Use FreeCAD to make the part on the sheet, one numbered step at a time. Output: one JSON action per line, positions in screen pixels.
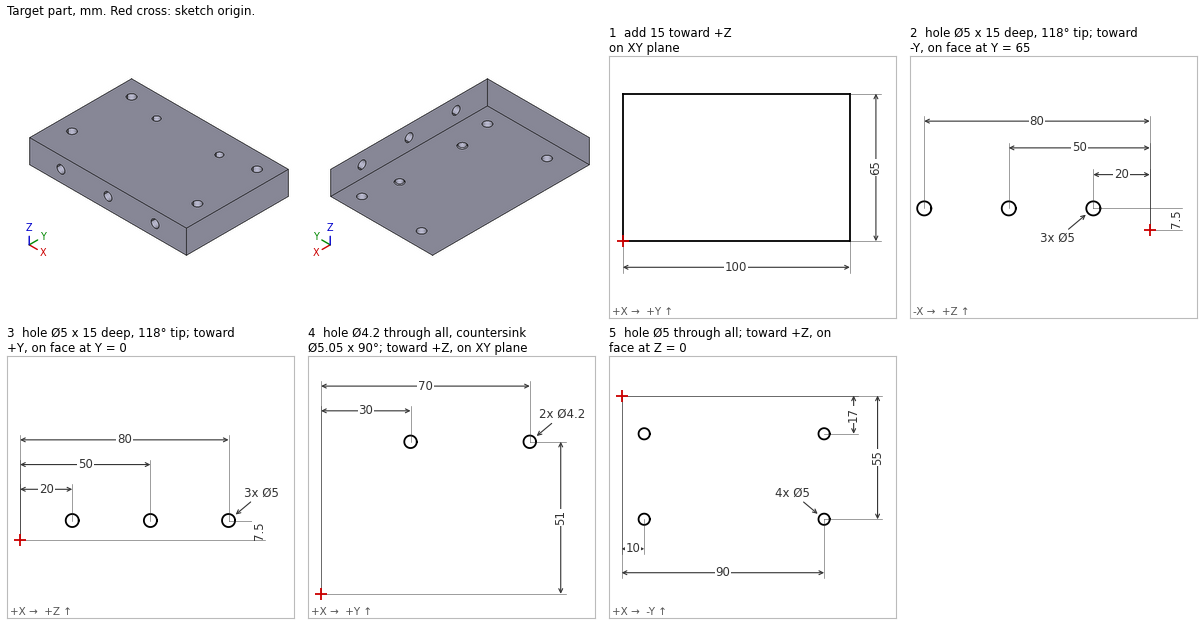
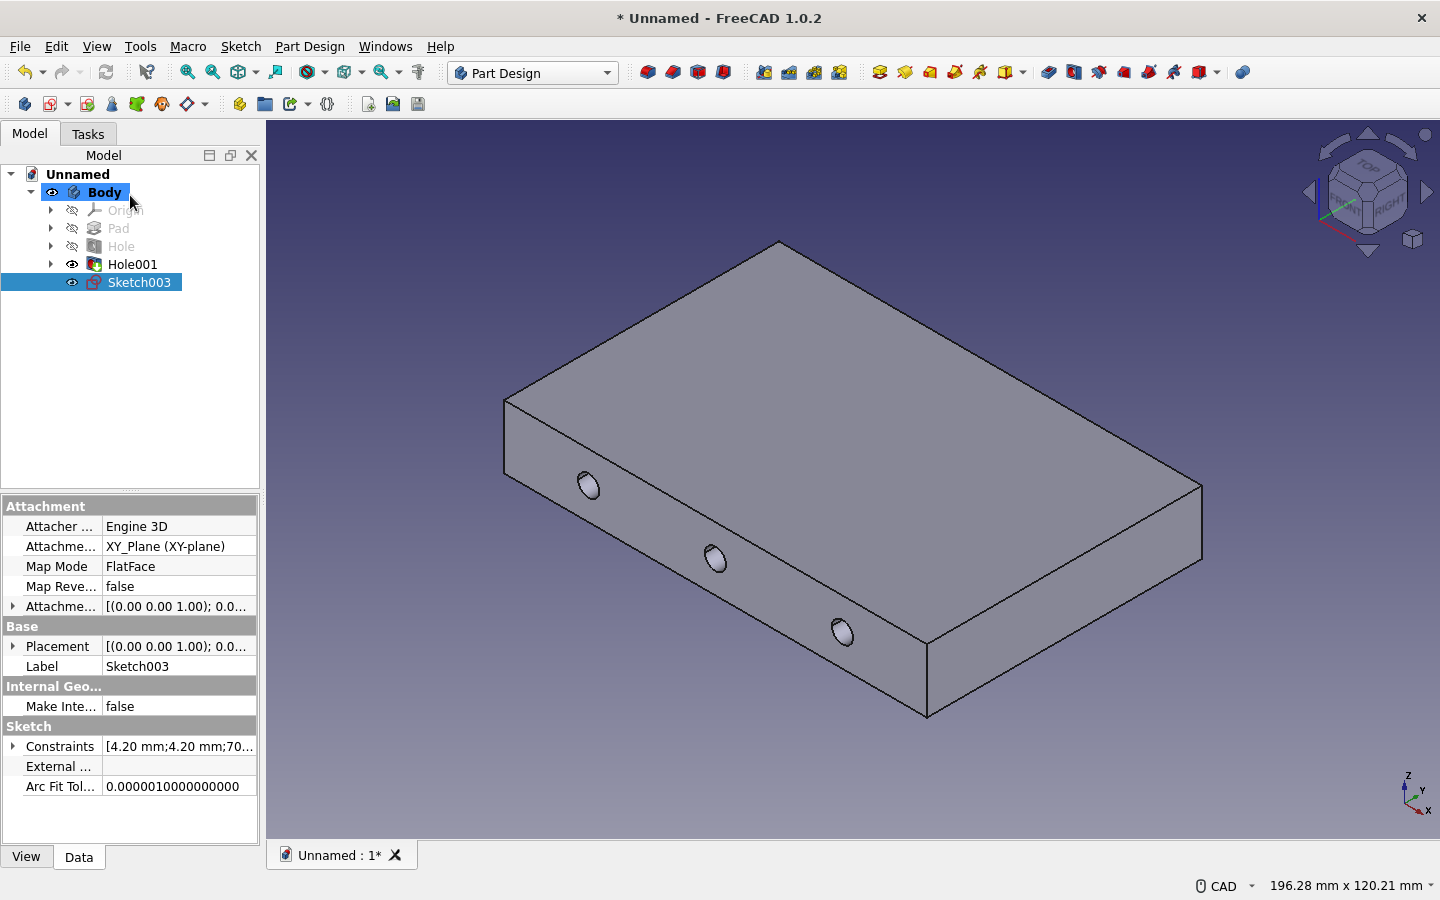
{"action": "left_click", "coordinate": [1074, 72]}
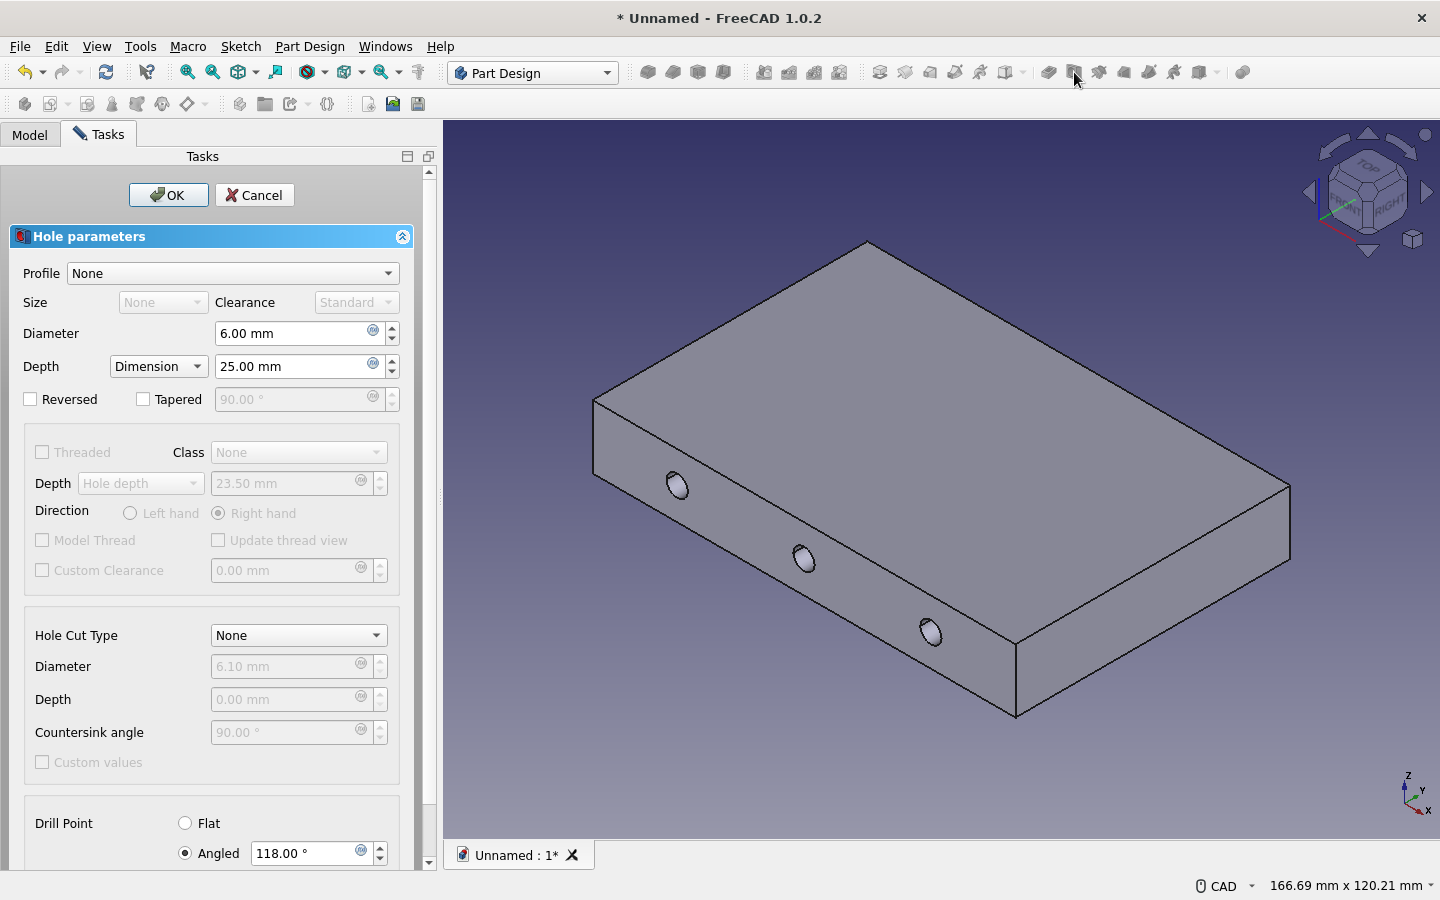
{"action": "triple_click", "coordinate": [300, 334]}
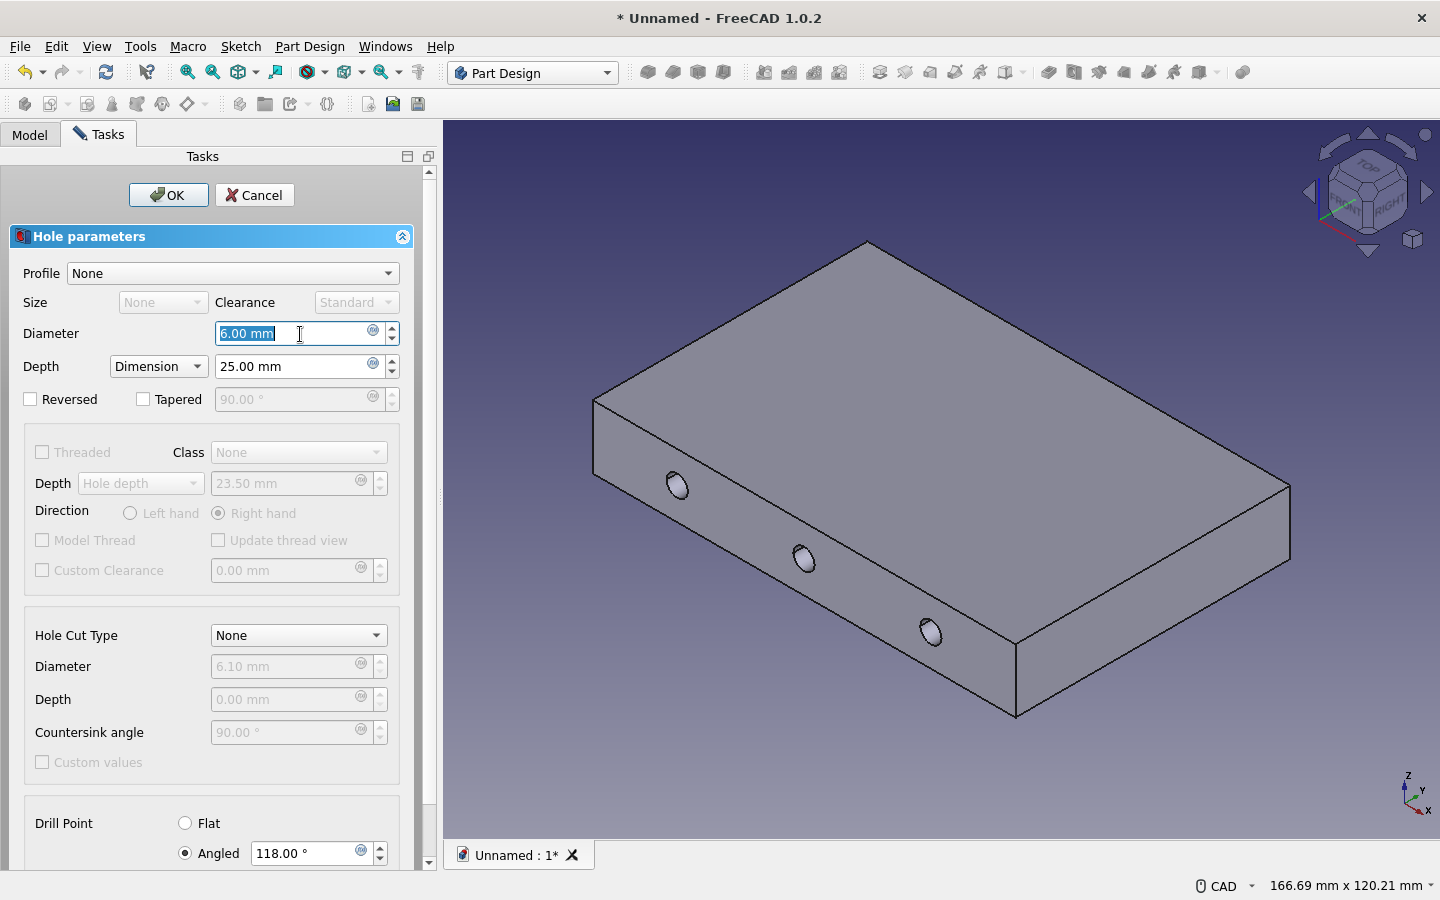
{"action": "type", "text": "4.2"}
{"action": "key", "text": "Tab"}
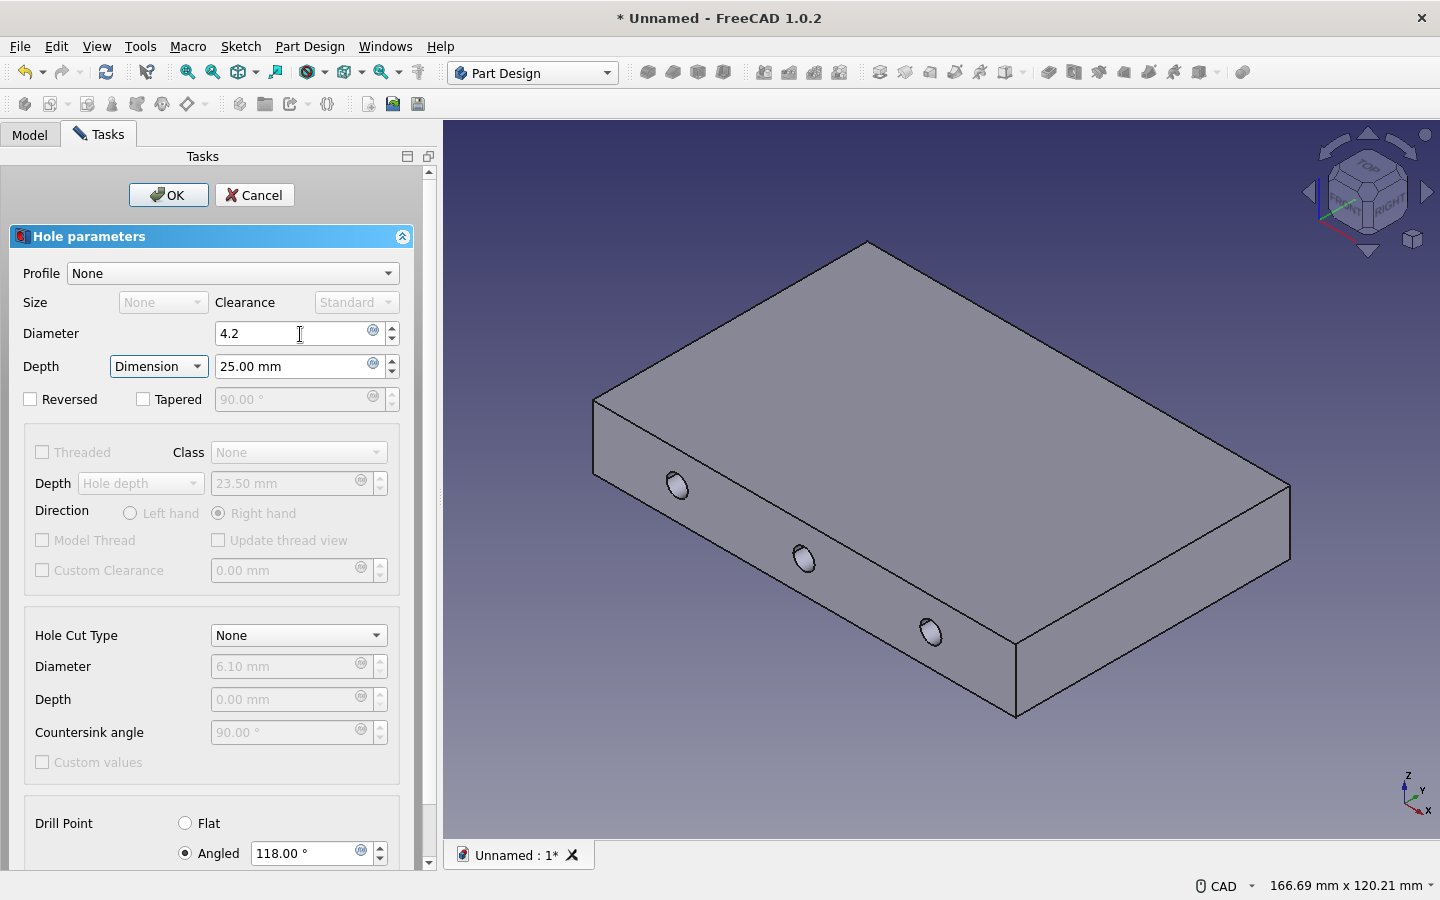
{"action": "left_click", "coordinate": [160, 366]}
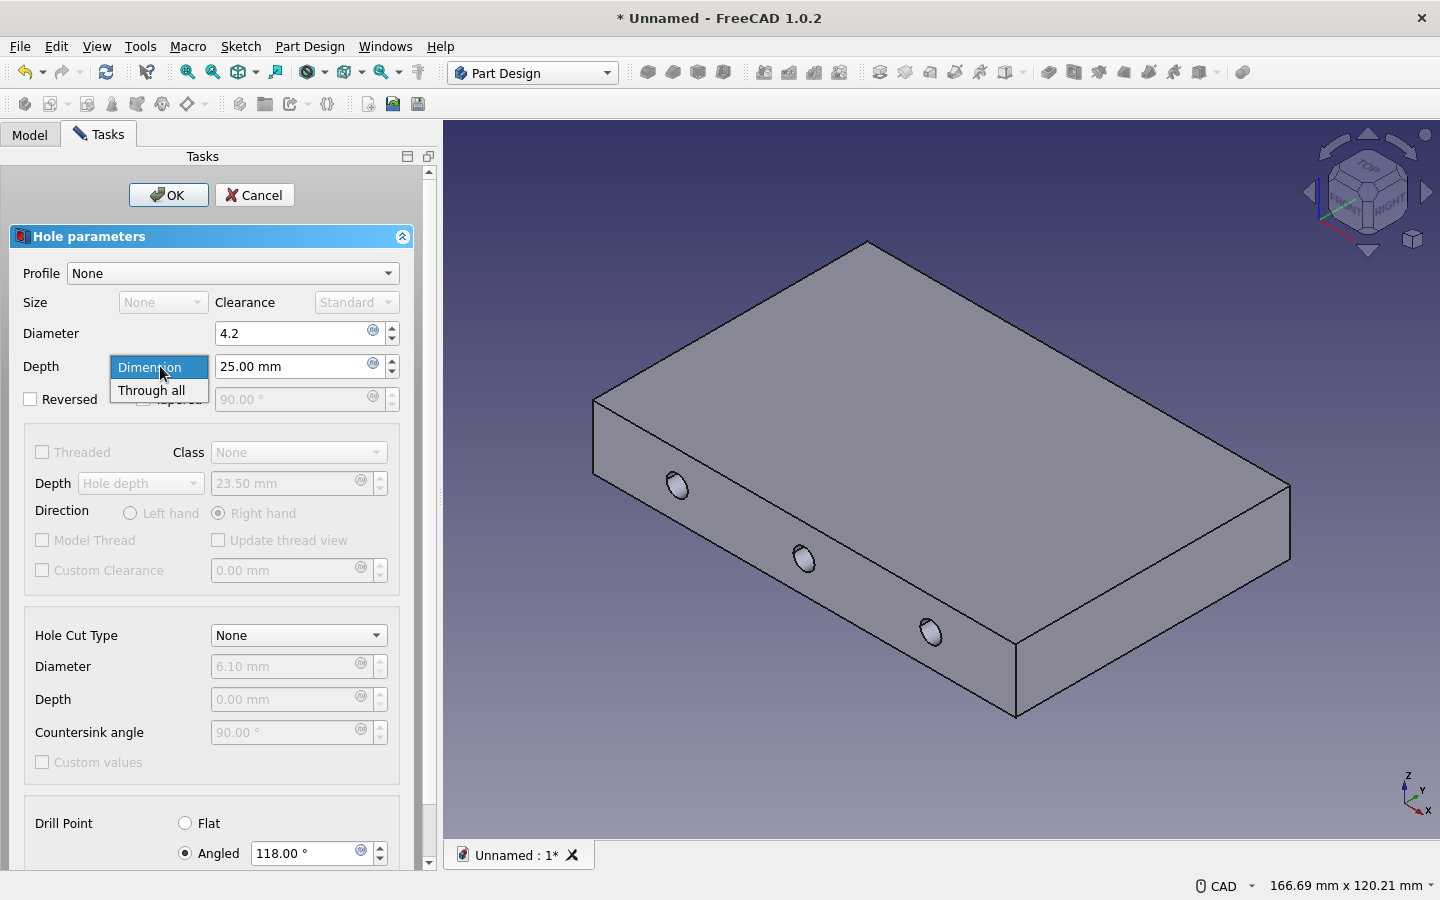
{"action": "left_click", "coordinate": [158, 390]}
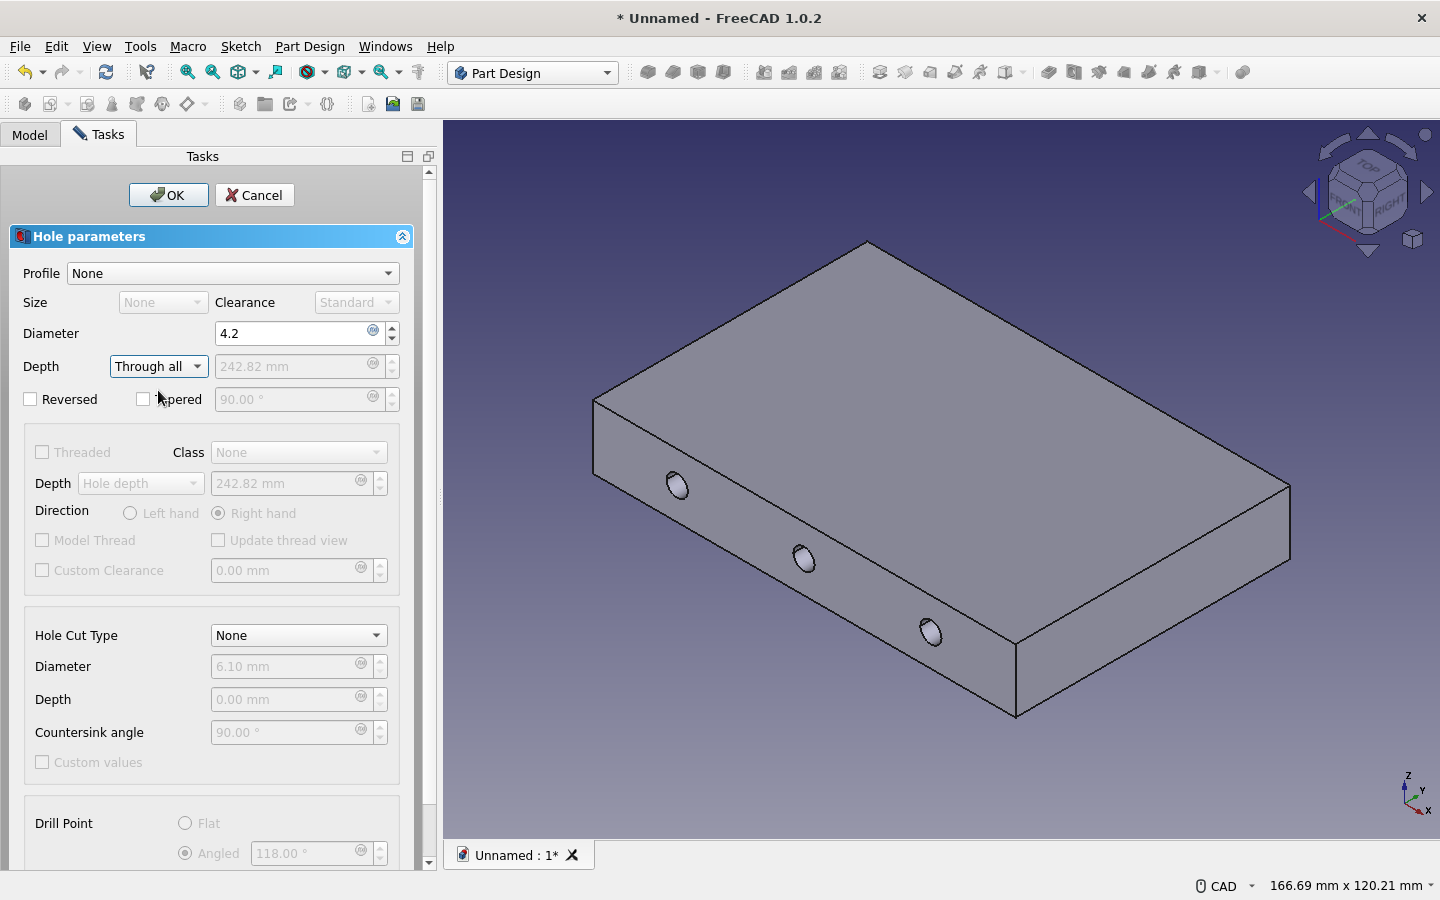
{"action": "left_click", "coordinate": [31, 399]}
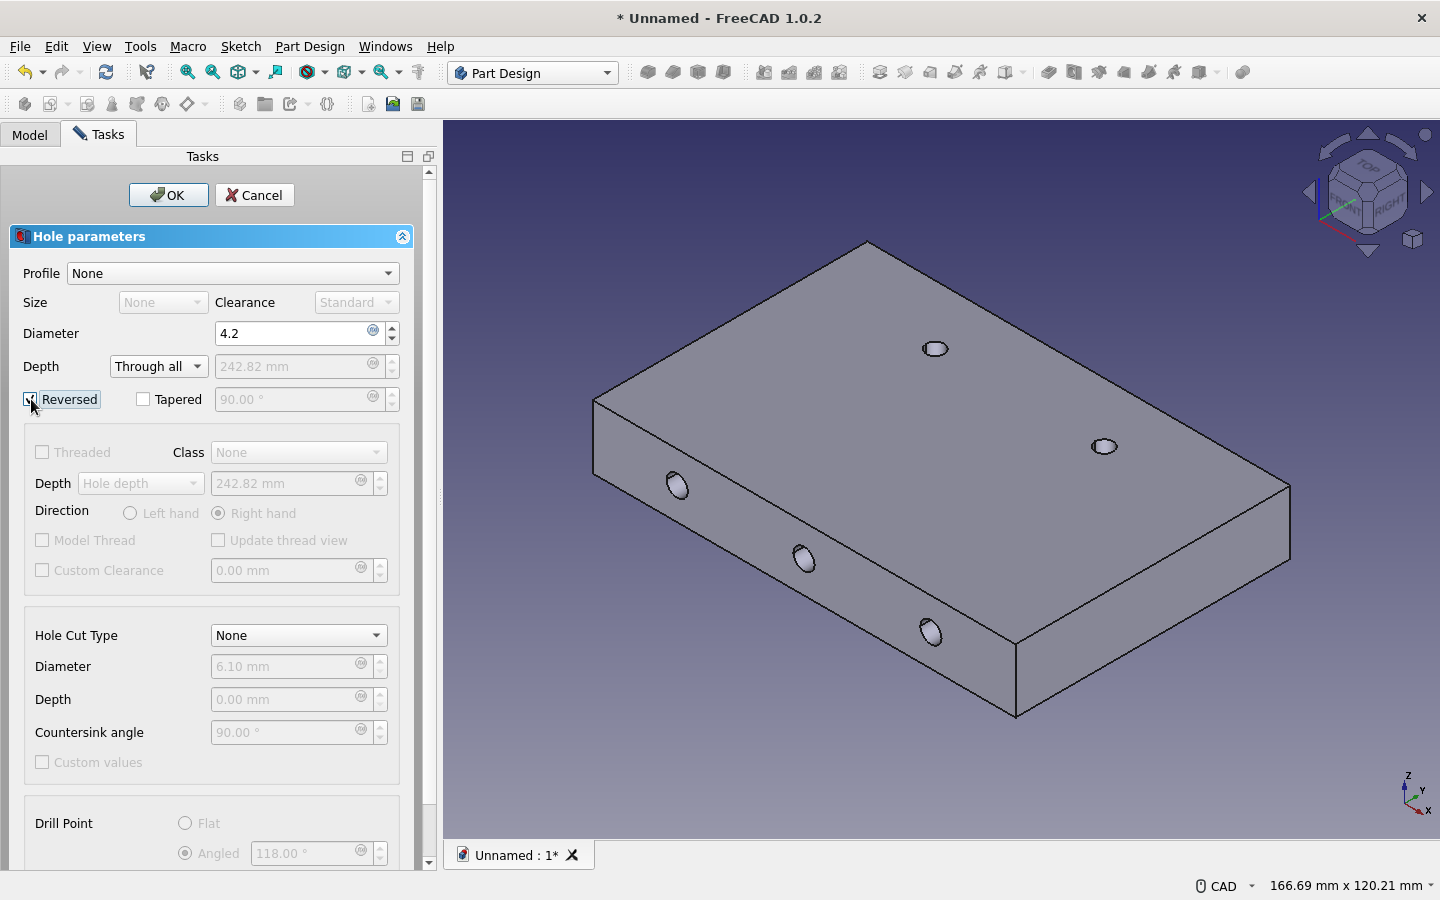
{"action": "left_click", "coordinate": [300, 636]}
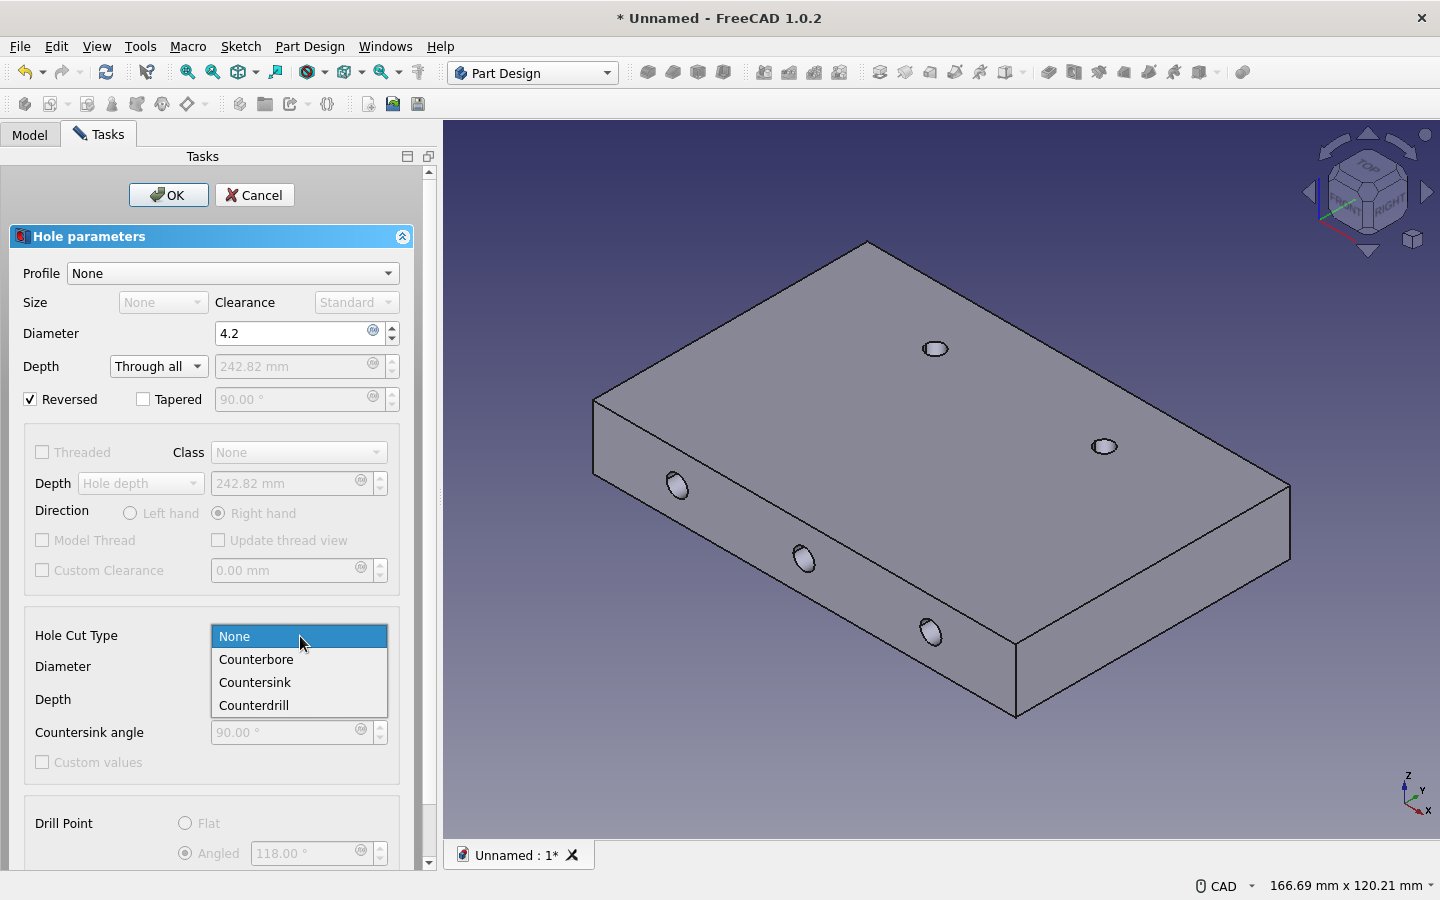
{"action": "left_click", "coordinate": [298, 682]}